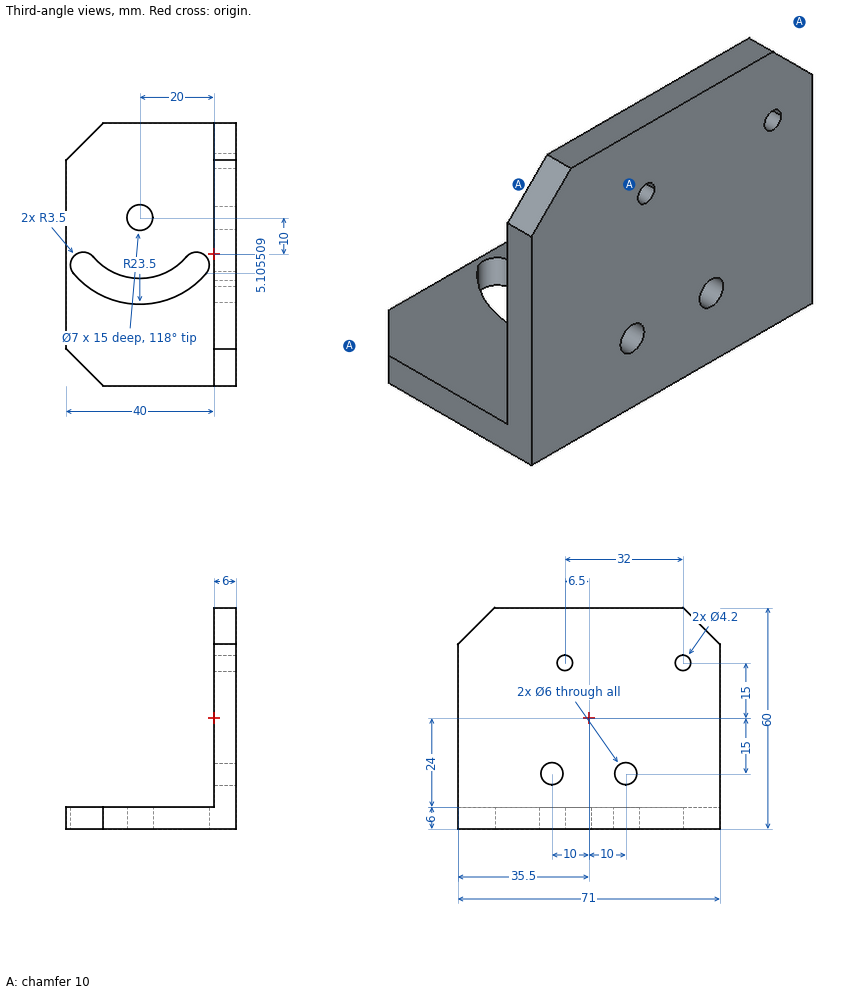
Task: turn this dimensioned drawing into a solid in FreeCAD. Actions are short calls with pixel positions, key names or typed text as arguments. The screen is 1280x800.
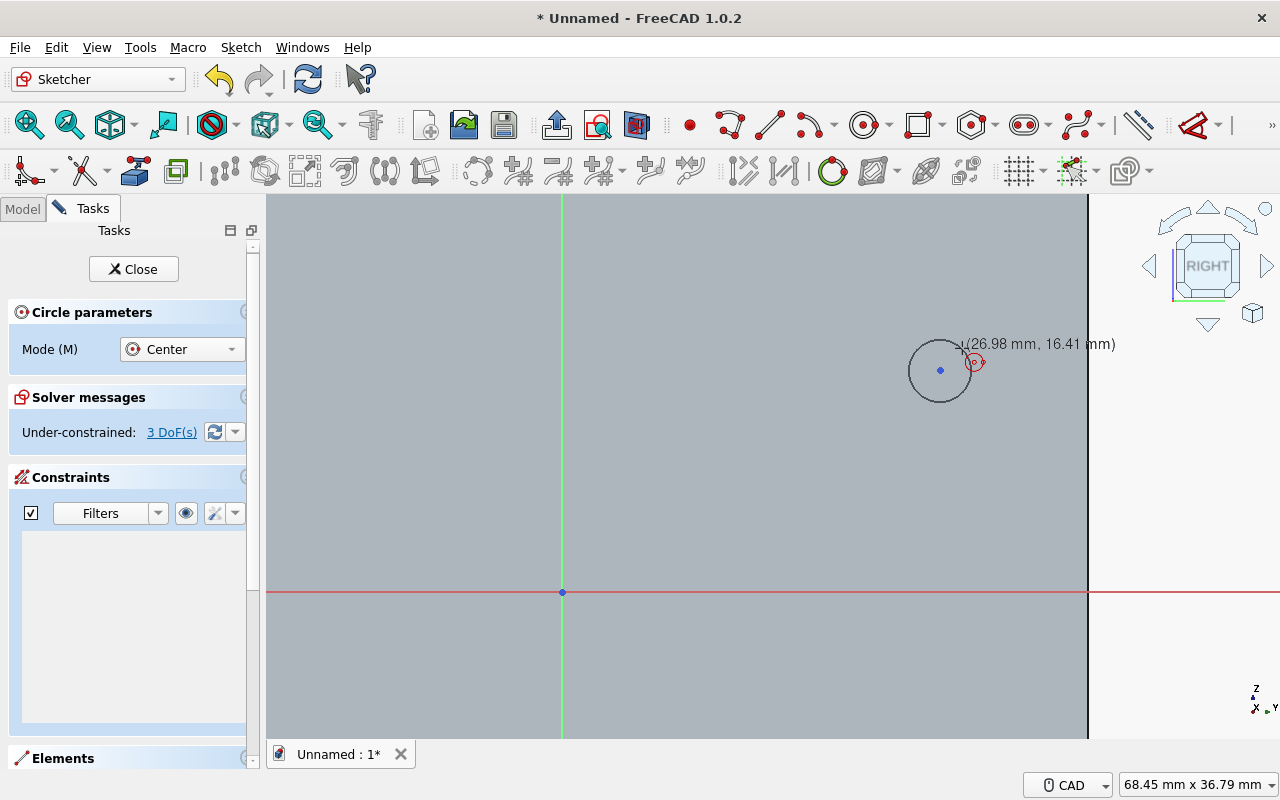
click(466, 370)
click(488, 348)
key(Escape)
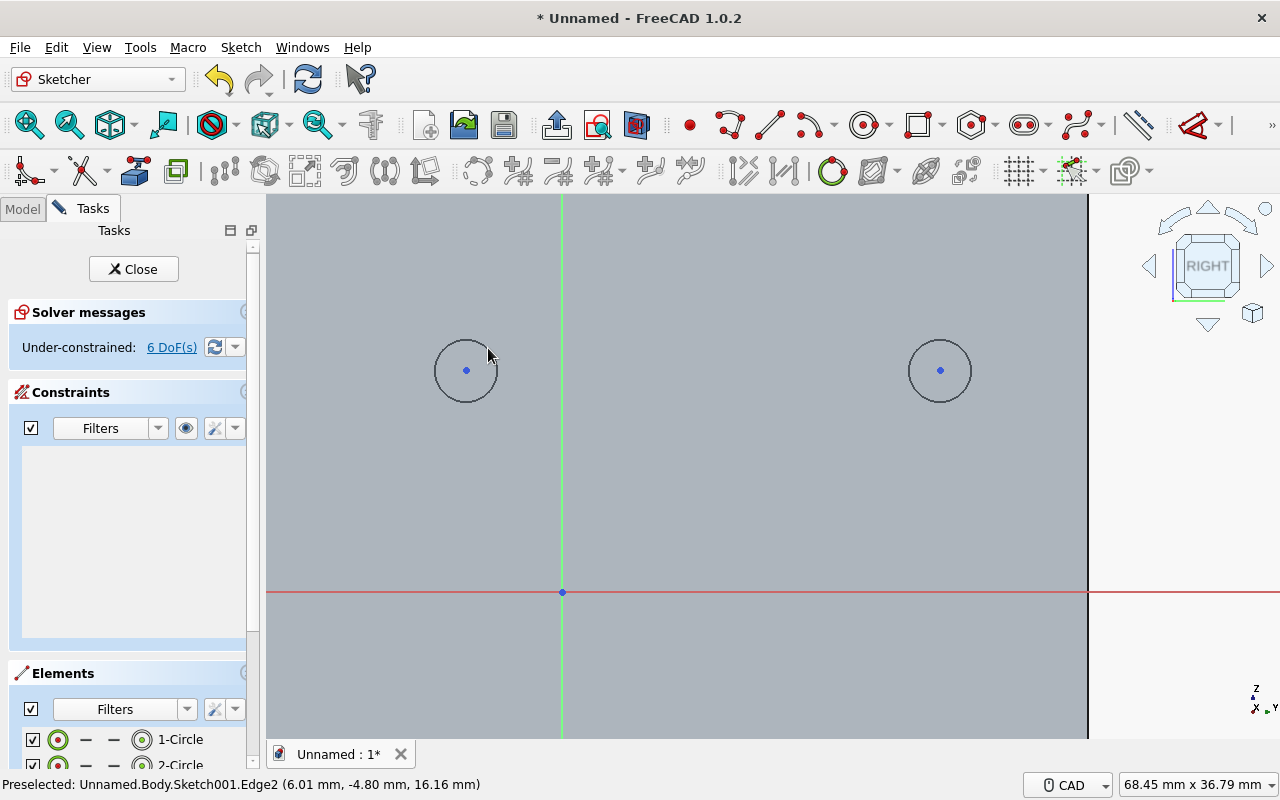
click(962, 349)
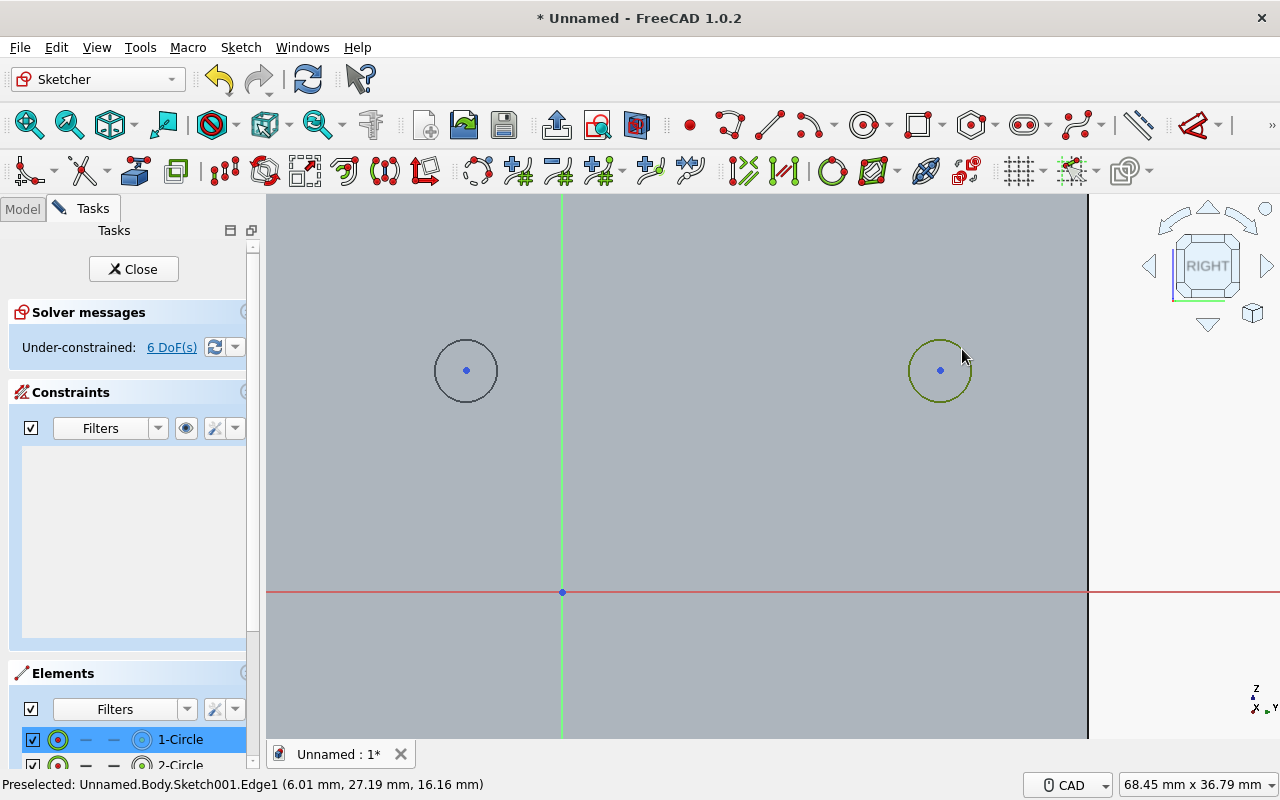
click(488, 349)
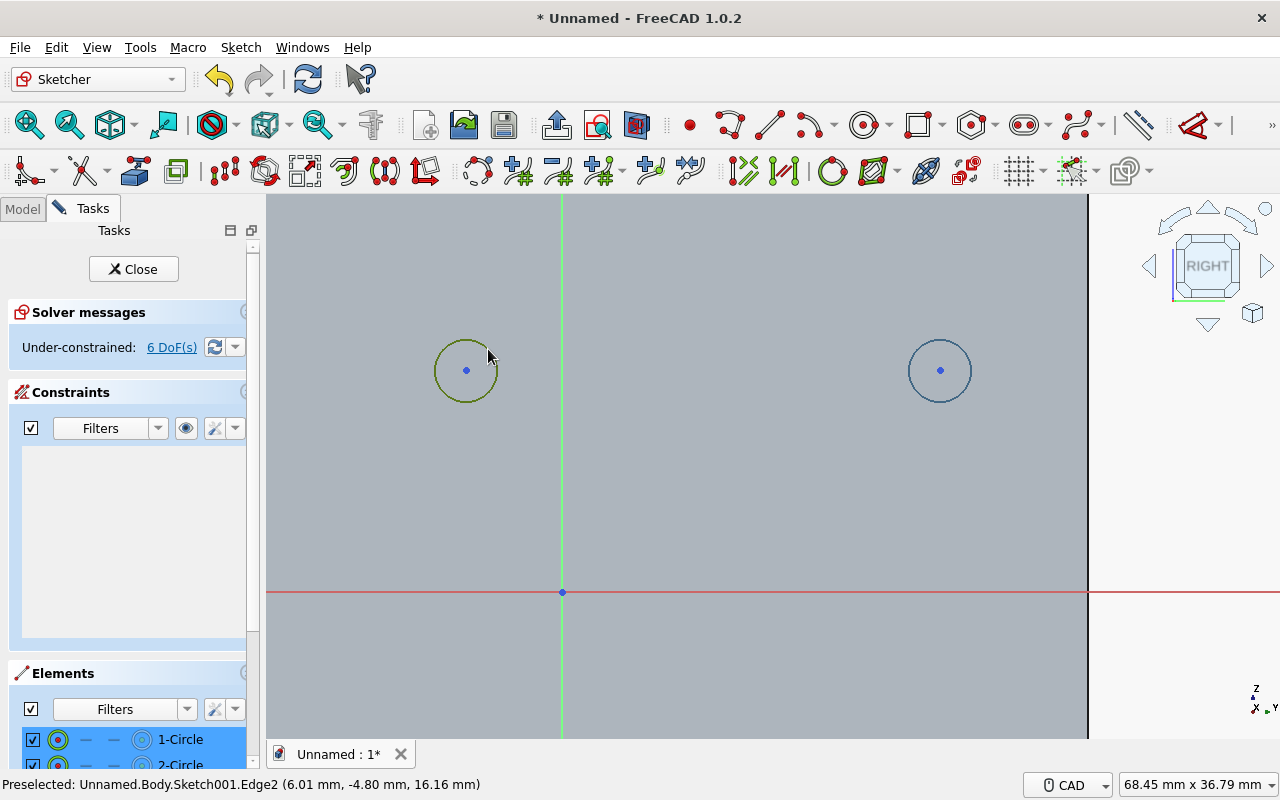
key(e)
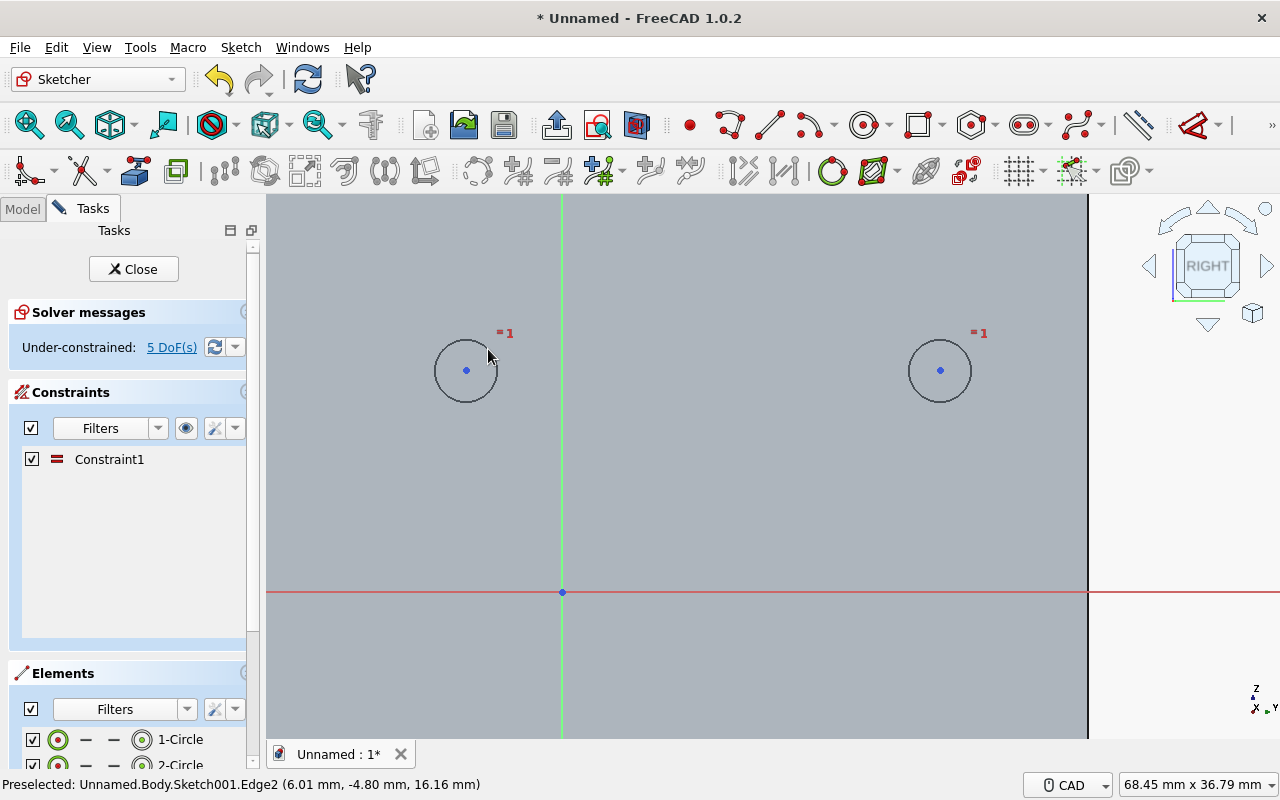
click(940, 371)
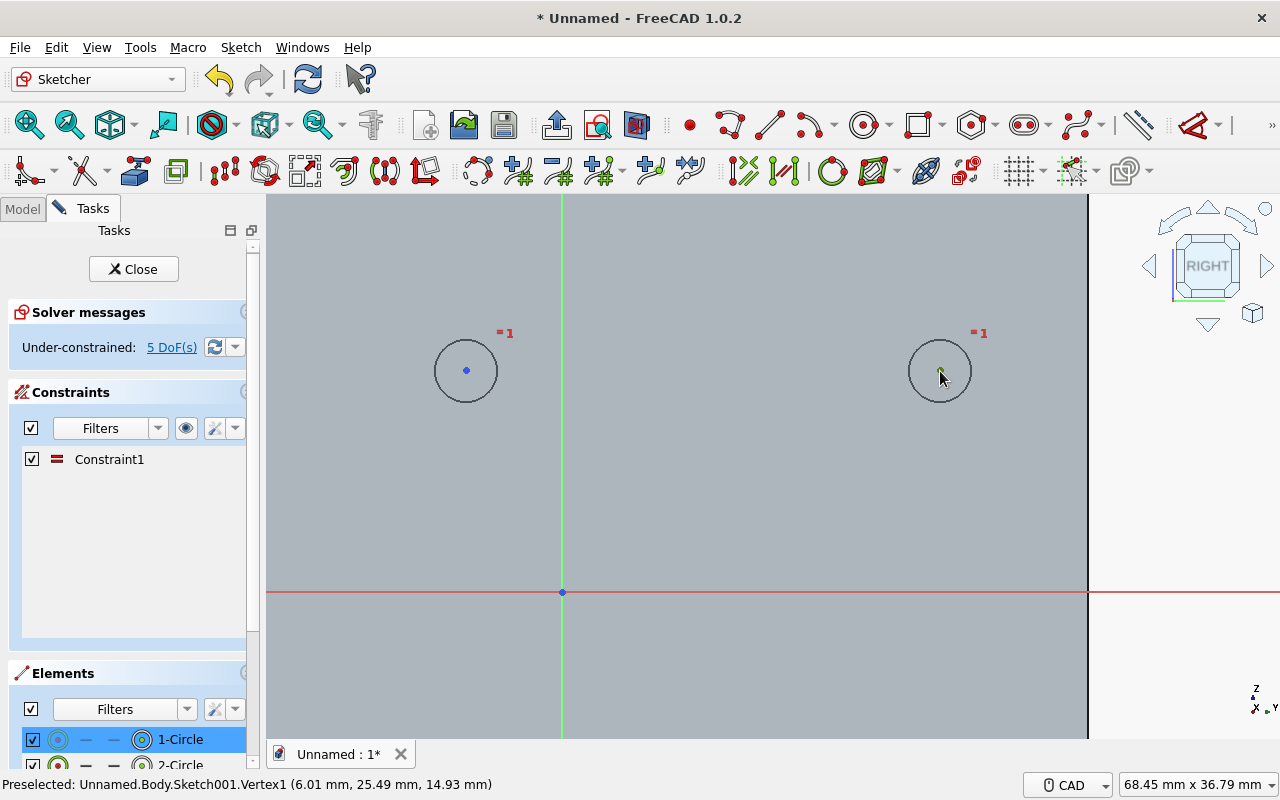
click(466, 371)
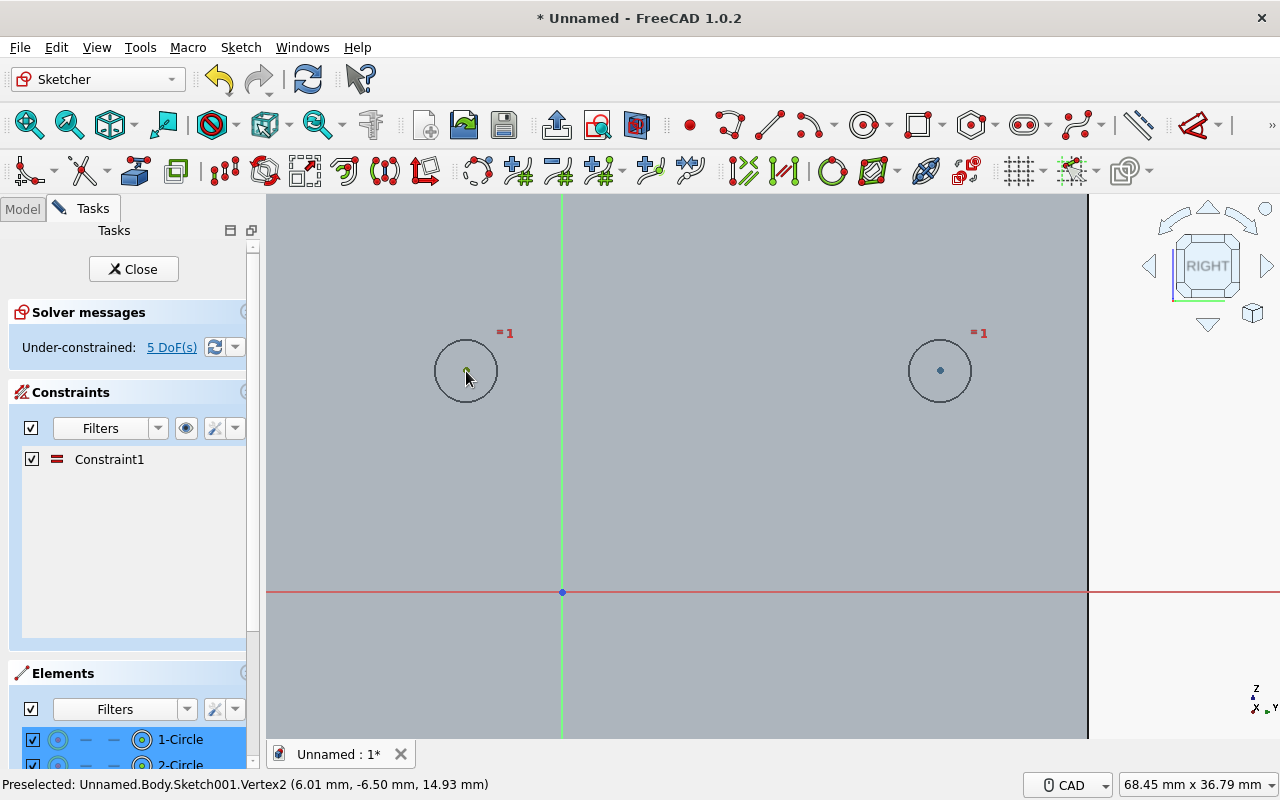
key(h)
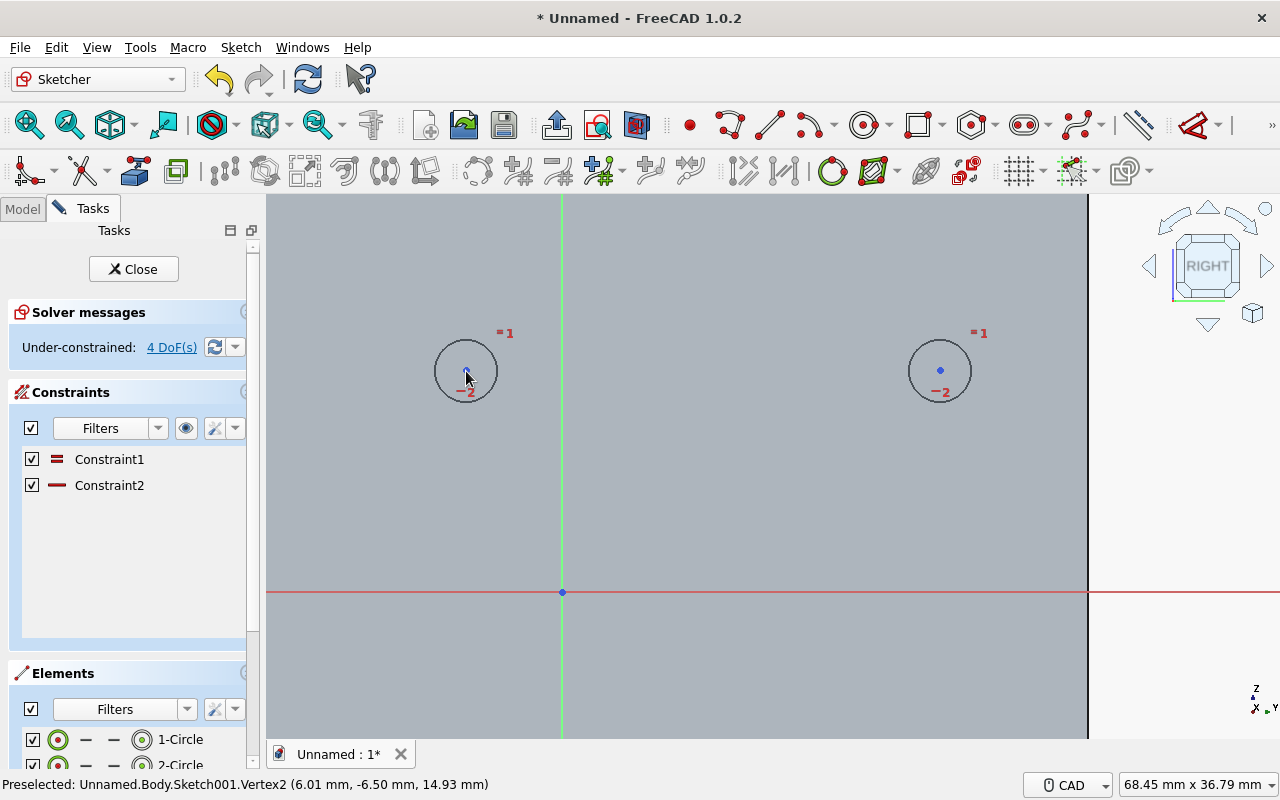
click(1194, 126)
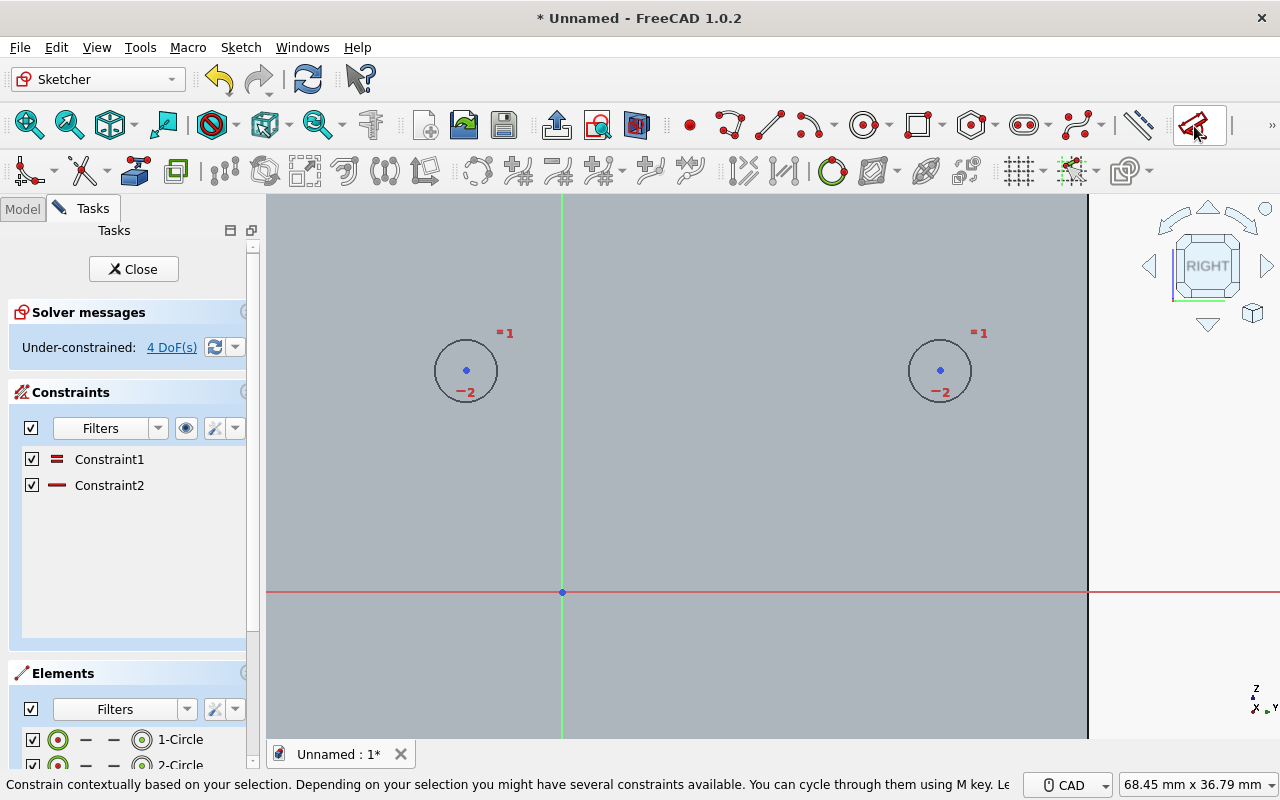
click(962, 349)
click(985, 326)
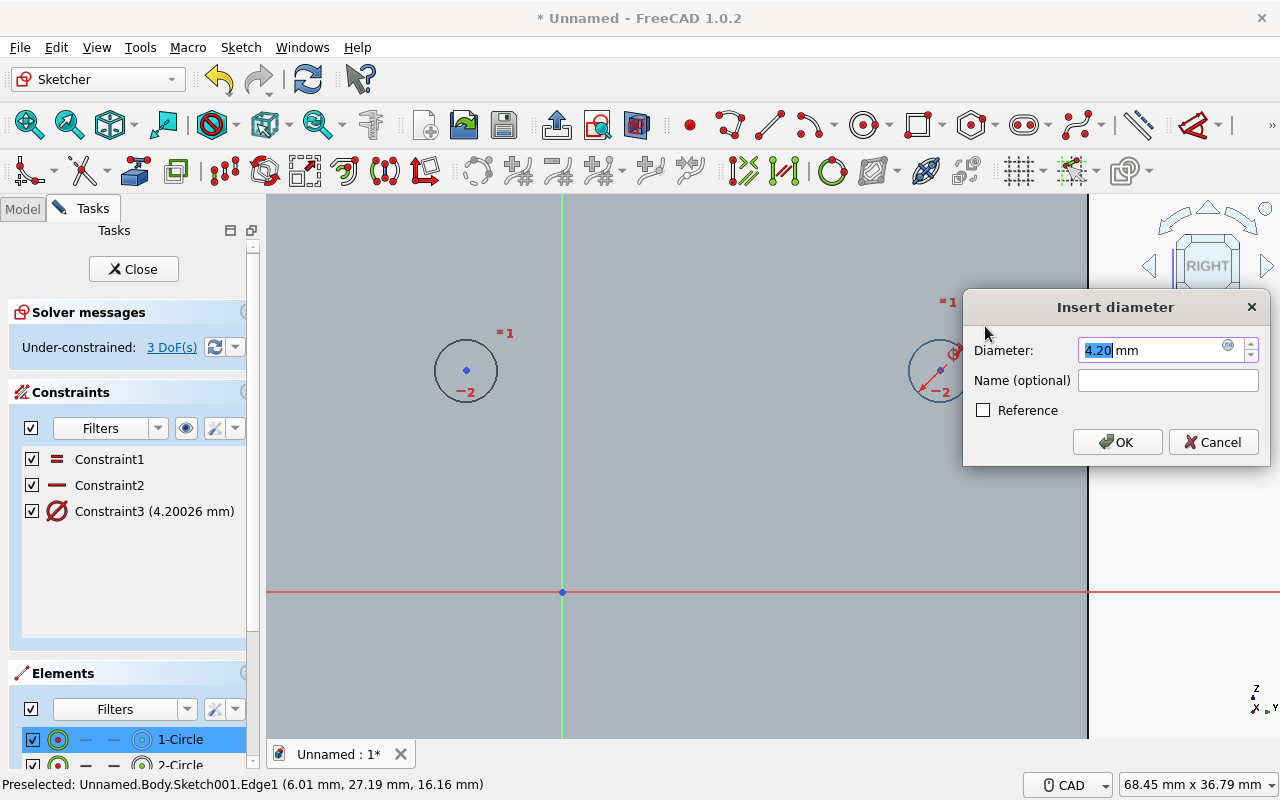
text(4.2)
key(Return)